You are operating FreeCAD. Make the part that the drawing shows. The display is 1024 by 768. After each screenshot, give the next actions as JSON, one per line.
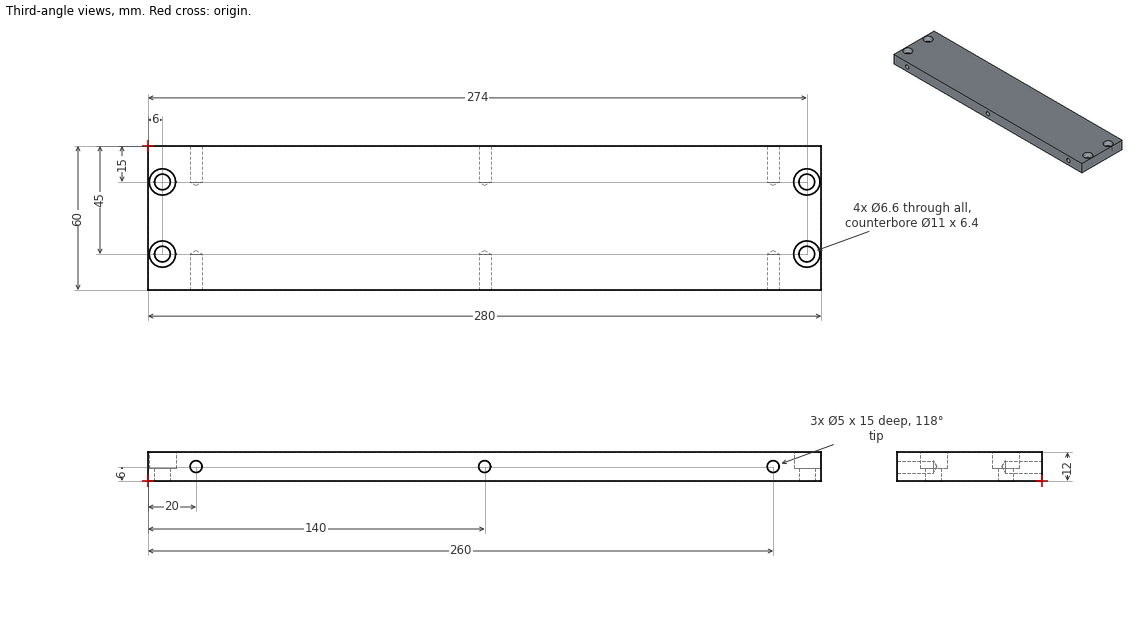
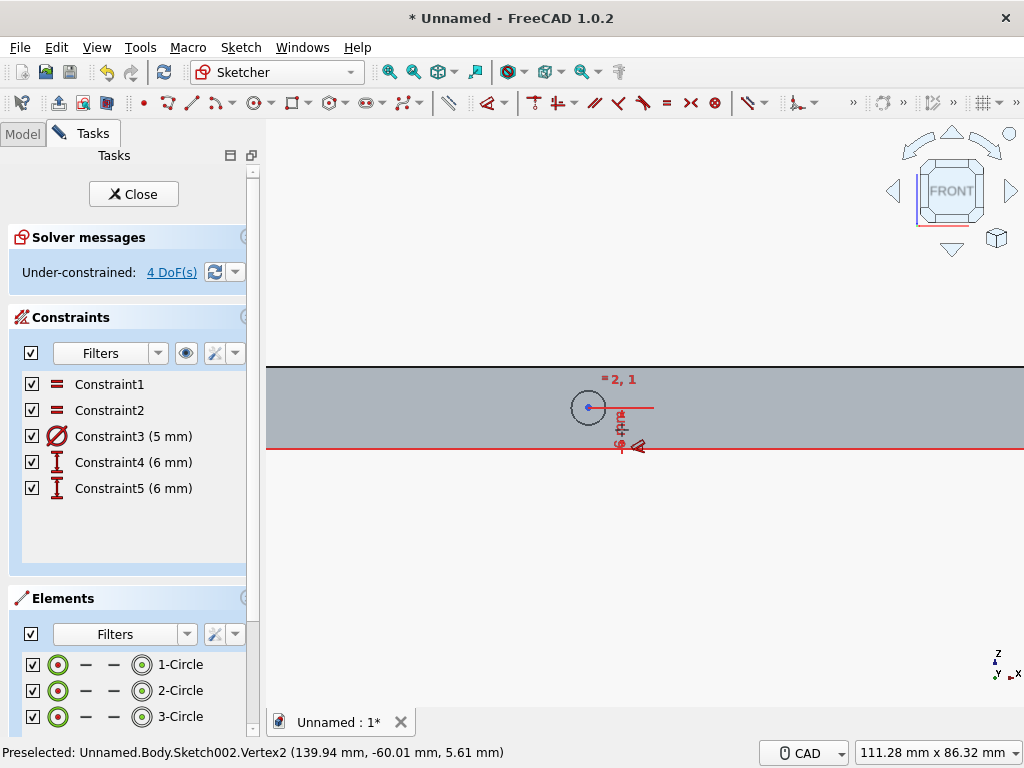
{"action": "scroll", "coordinate": [588, 411], "scroll_direction": "down", "scroll_amount": 8}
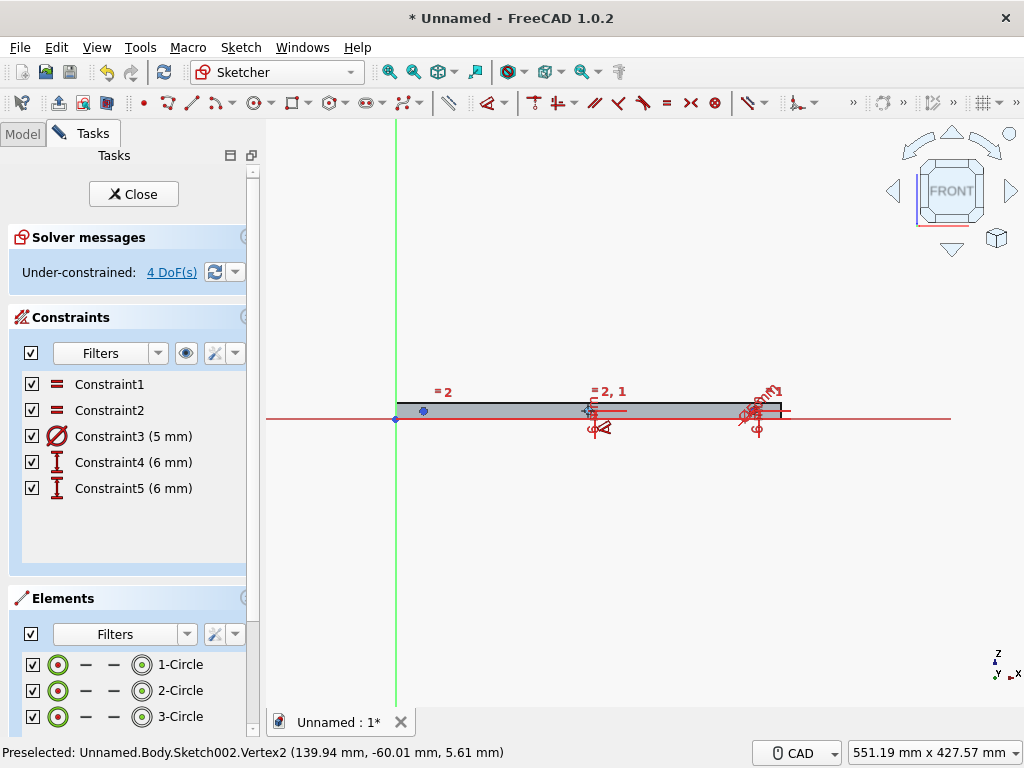
{"action": "scroll", "coordinate": [424, 411], "scroll_direction": "up", "scroll_amount": 8}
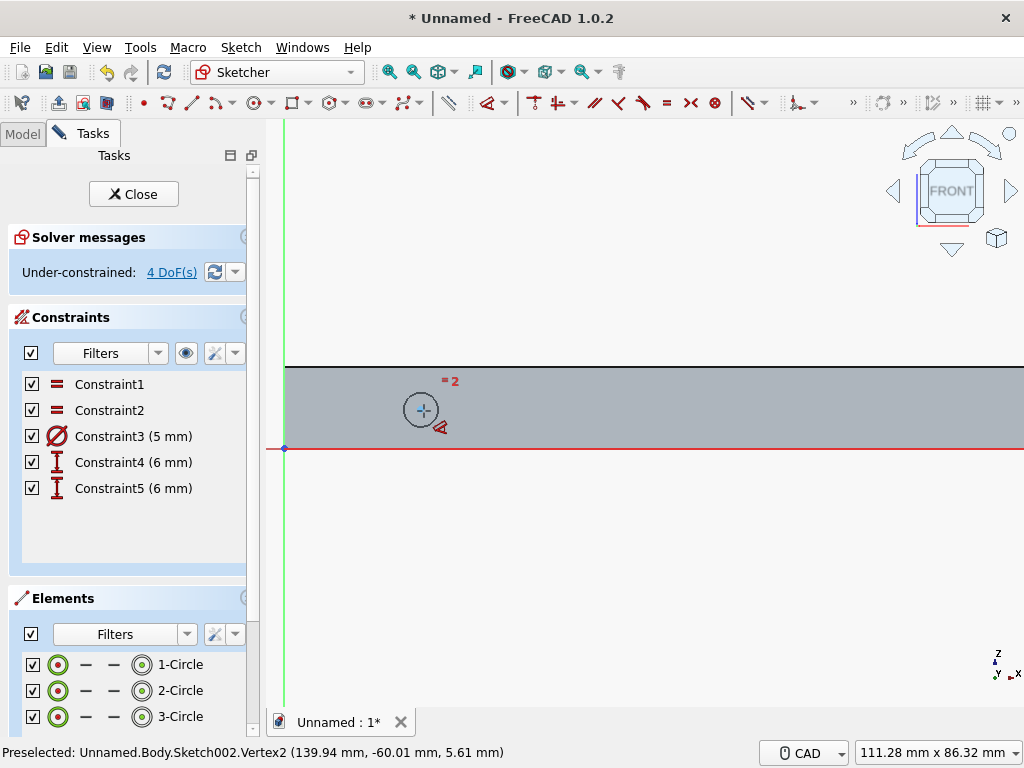
{"action": "left_click", "coordinate": [421, 410]}
{"action": "left_click", "coordinate": [455, 429]}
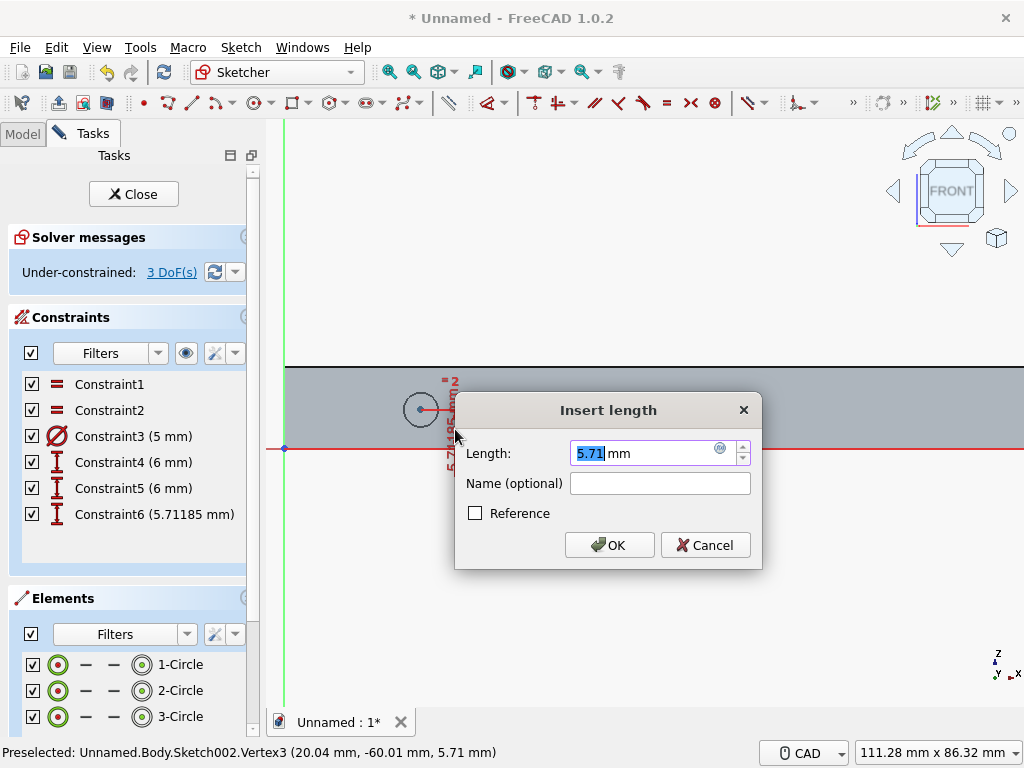
{"action": "type", "text": "6"}
{"action": "key", "text": "Return"}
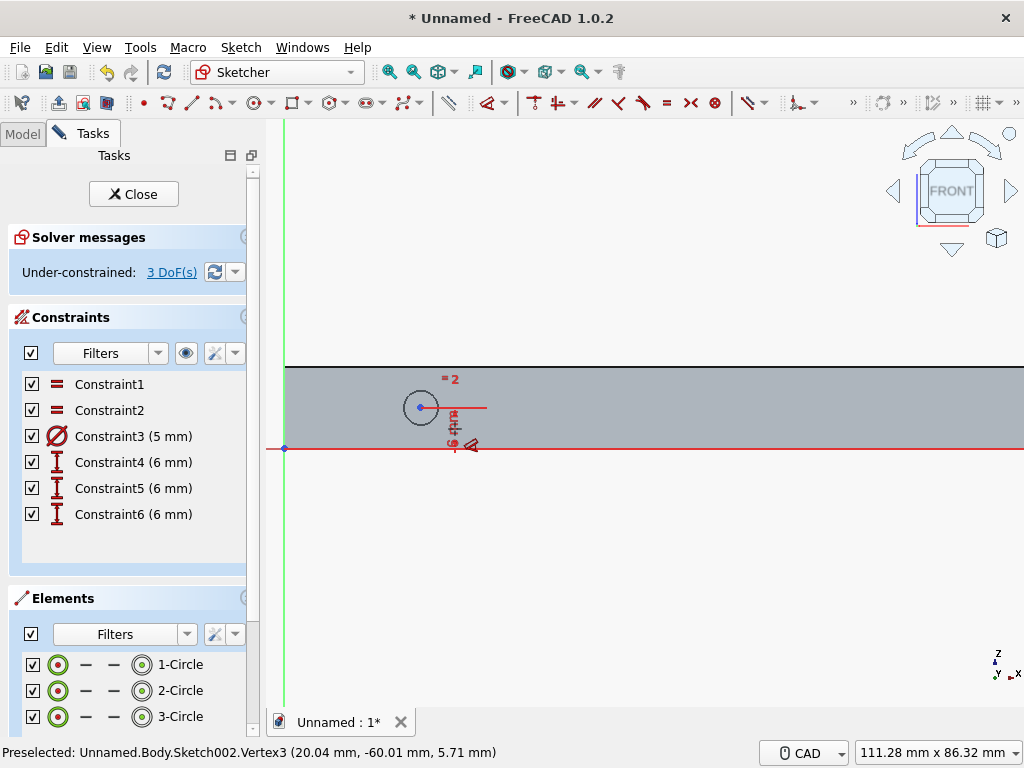
{"action": "scroll", "coordinate": [424, 411], "scroll_direction": "down", "scroll_amount": 8}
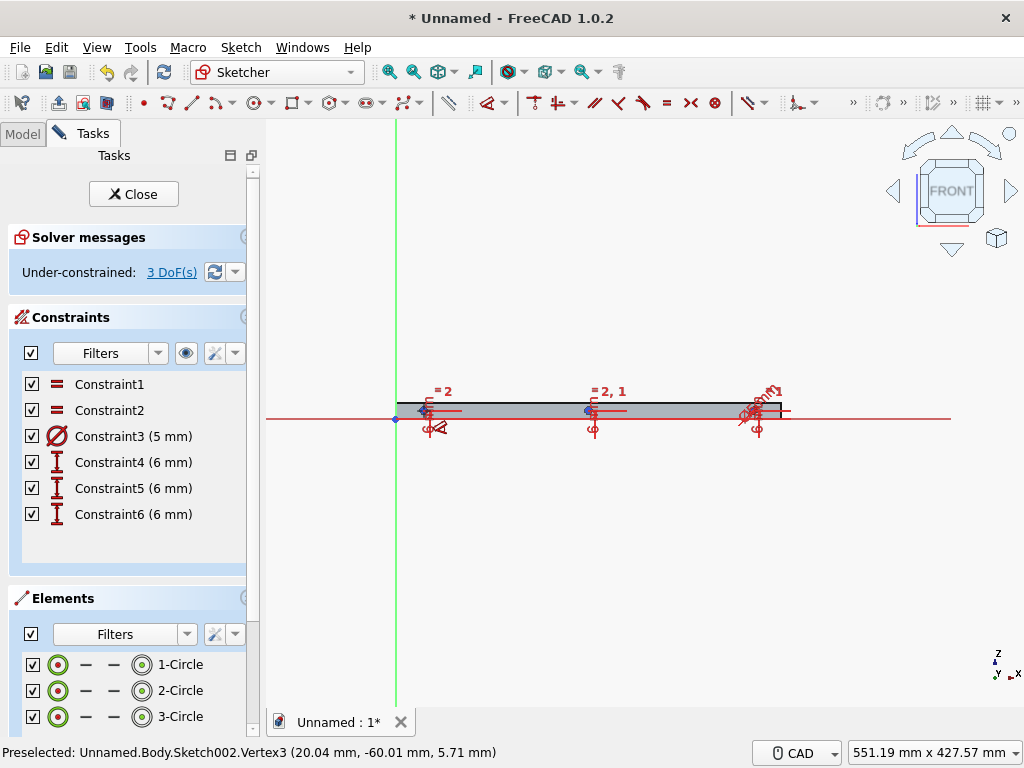
{"action": "scroll", "coordinate": [424, 411], "scroll_direction": "up", "scroll_amount": 2}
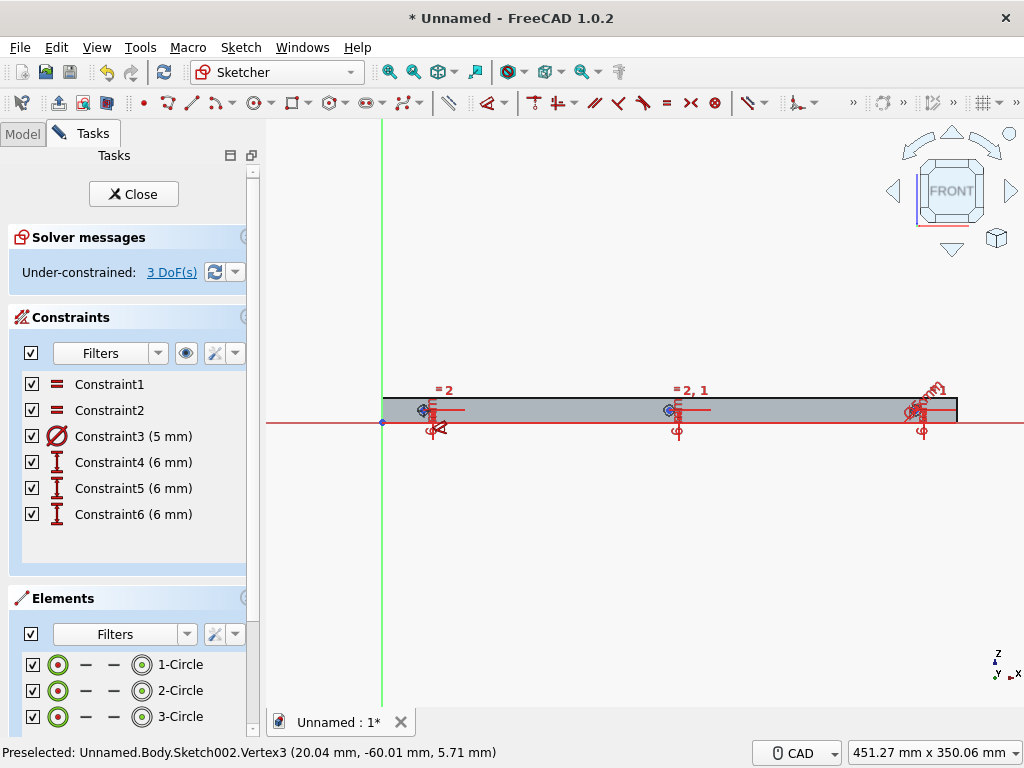
{"action": "left_click", "coordinate": [423, 410]}
{"action": "left_click", "coordinate": [403, 457]}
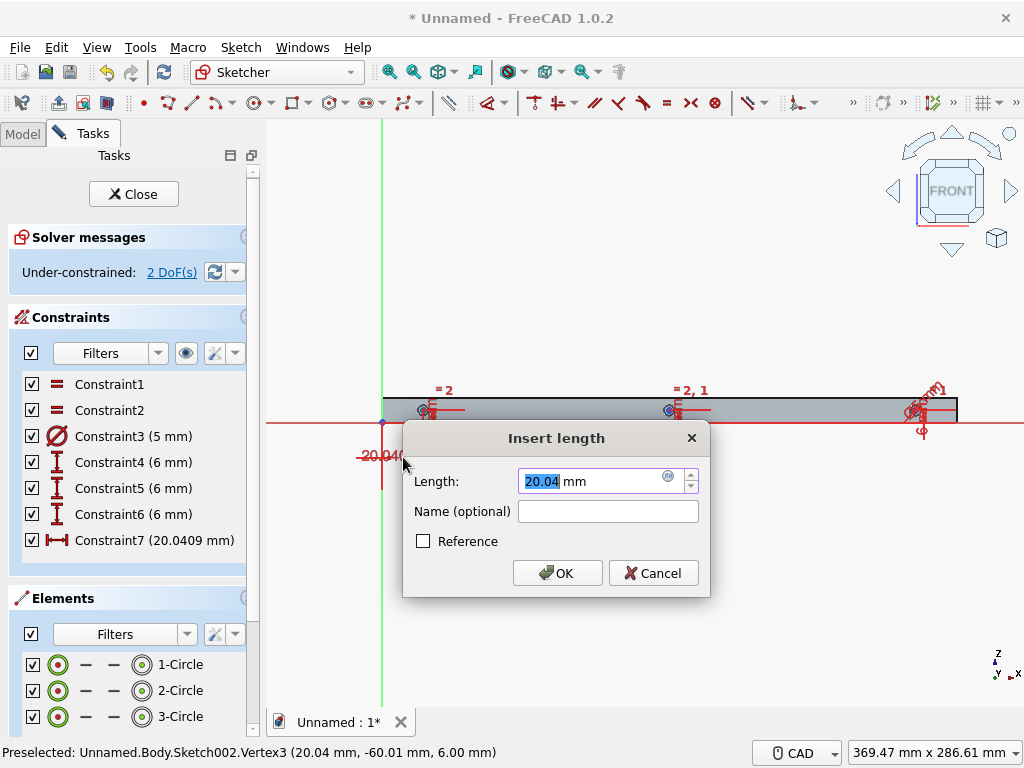
{"action": "type", "text": "20"}
{"action": "key", "text": "Return"}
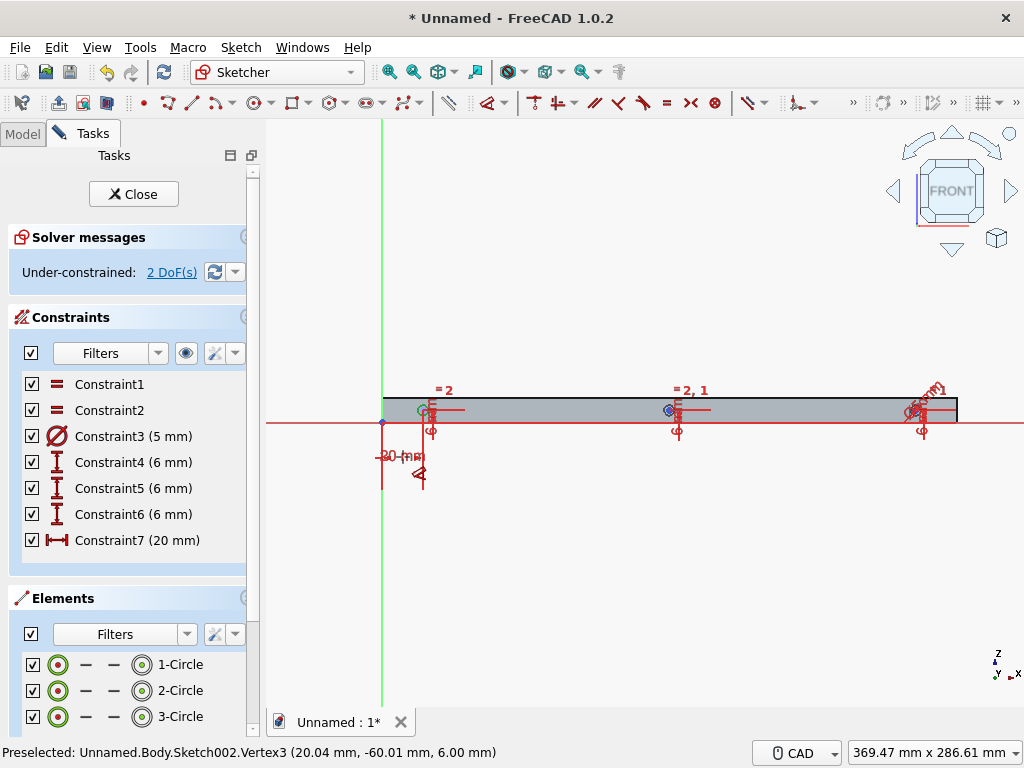
{"action": "scroll", "coordinate": [424, 411], "scroll_direction": "down", "scroll_amount": 2}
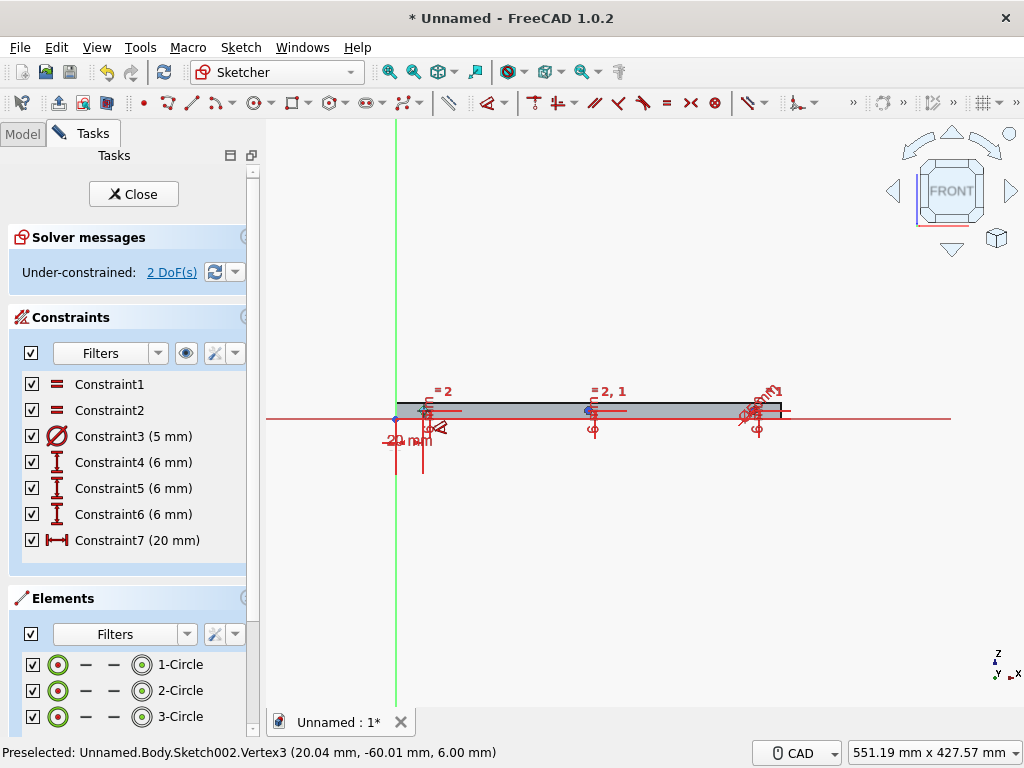
{"action": "left_click", "coordinate": [754, 411]}
{"action": "left_click", "coordinate": [575, 453]}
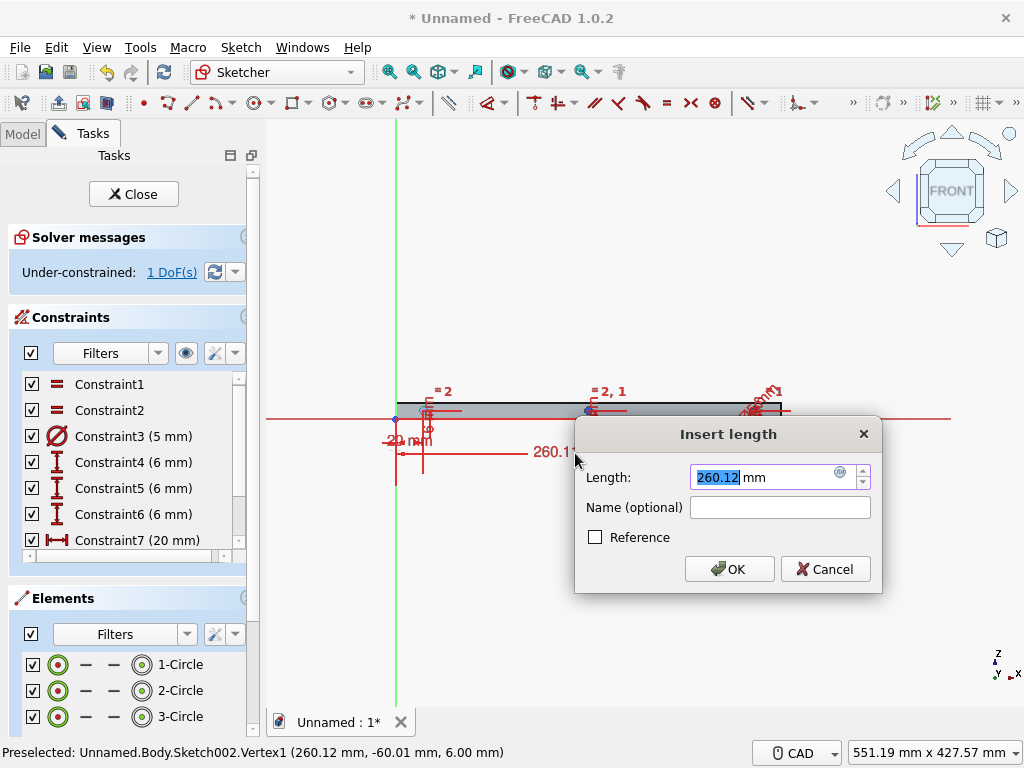
{"action": "type", "text": "260"}
{"action": "key", "text": "Return"}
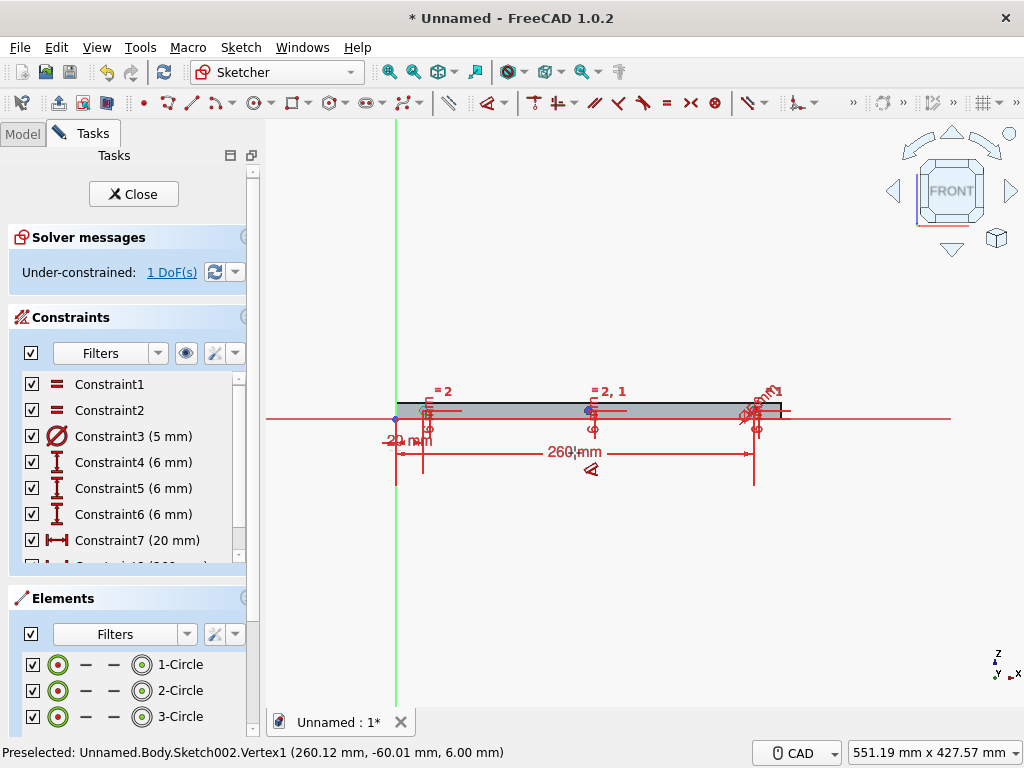
{"action": "left_click", "coordinate": [588, 411]}
{"action": "left_click", "coordinate": [492, 453]}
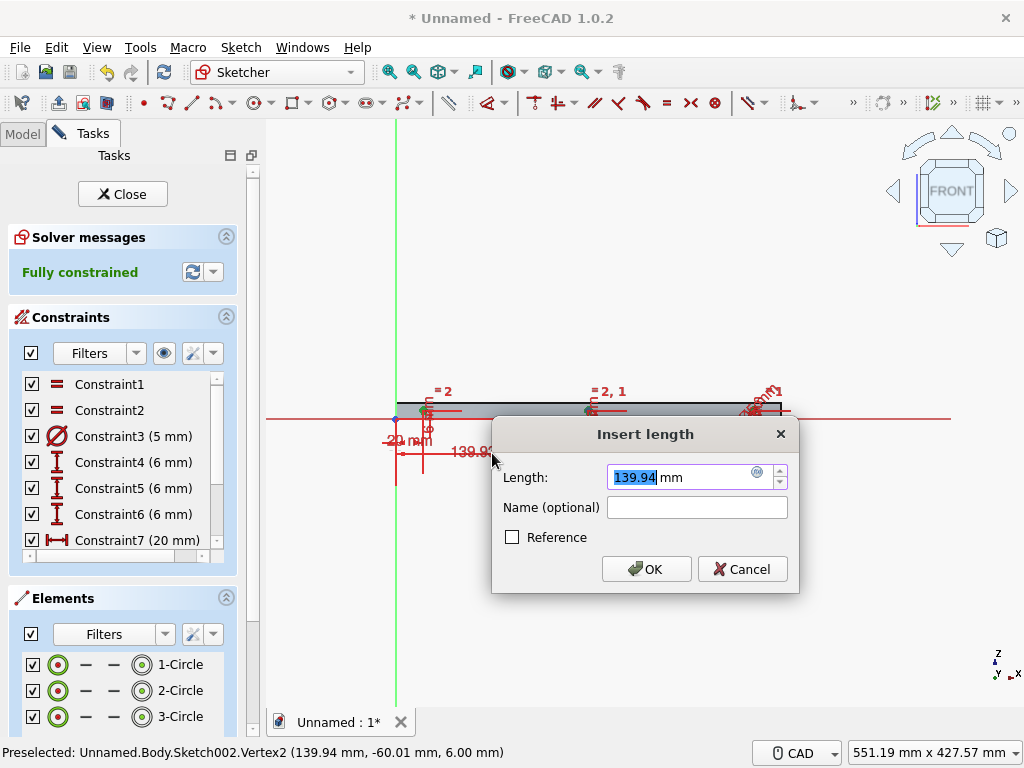
{"action": "type", "text": "140"}
{"action": "key", "text": "Return"}
{"action": "key", "text": "Escape"}